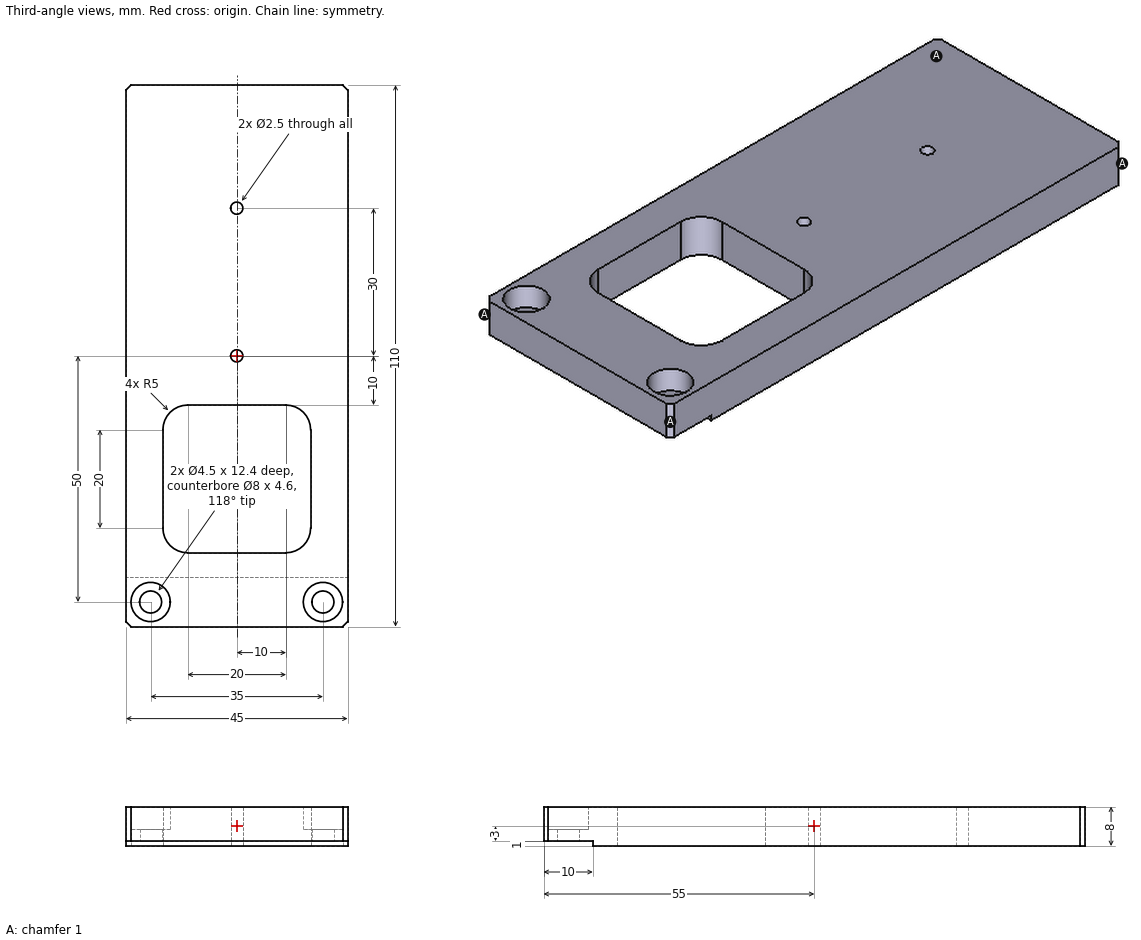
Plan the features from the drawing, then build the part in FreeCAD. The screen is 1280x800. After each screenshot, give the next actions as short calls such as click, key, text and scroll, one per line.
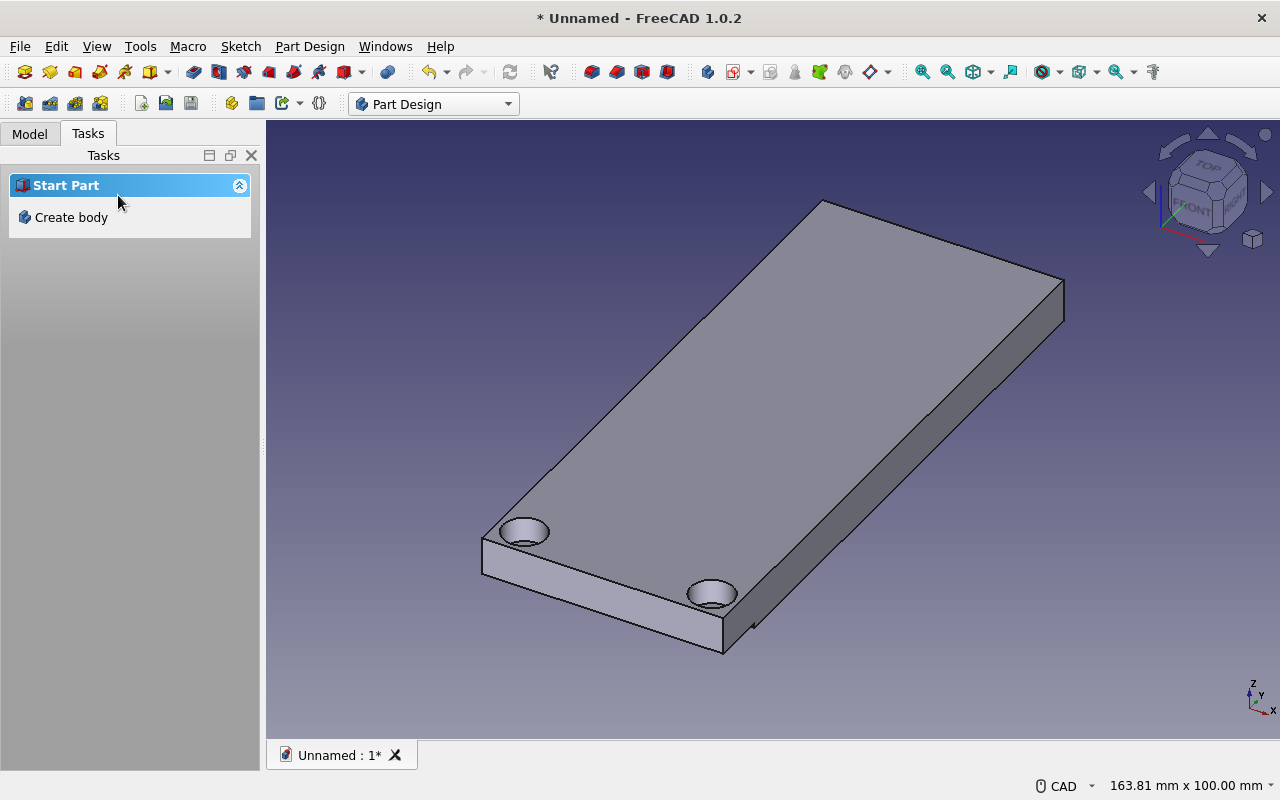
click(870, 312)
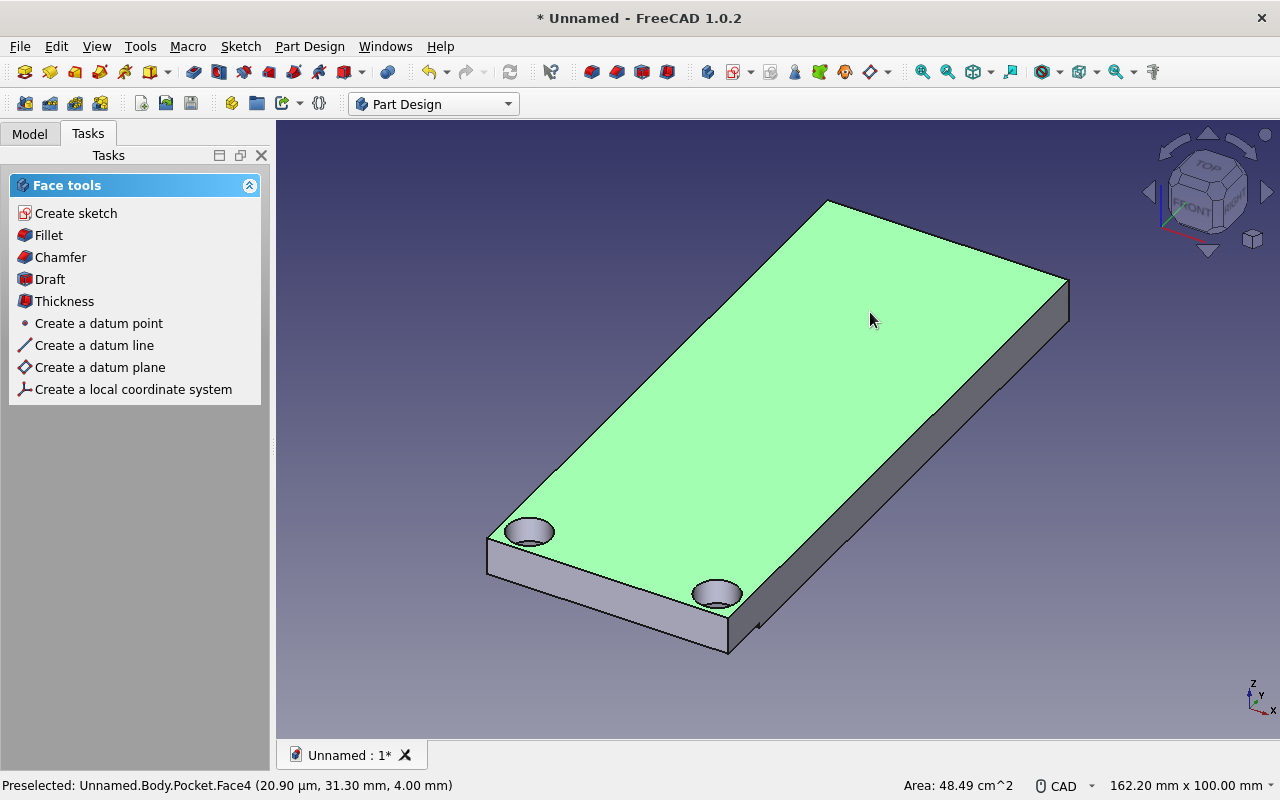
click(732, 72)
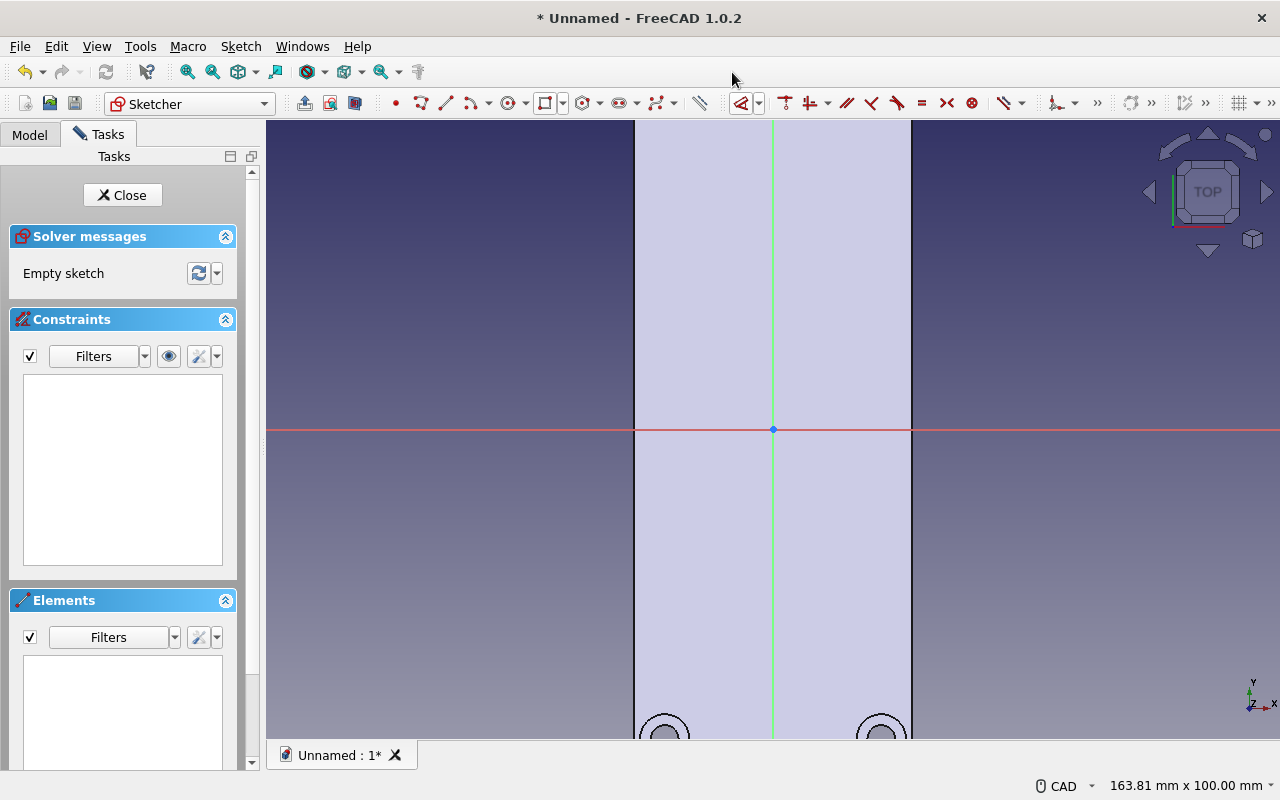
scroll(856, 224, up, 3)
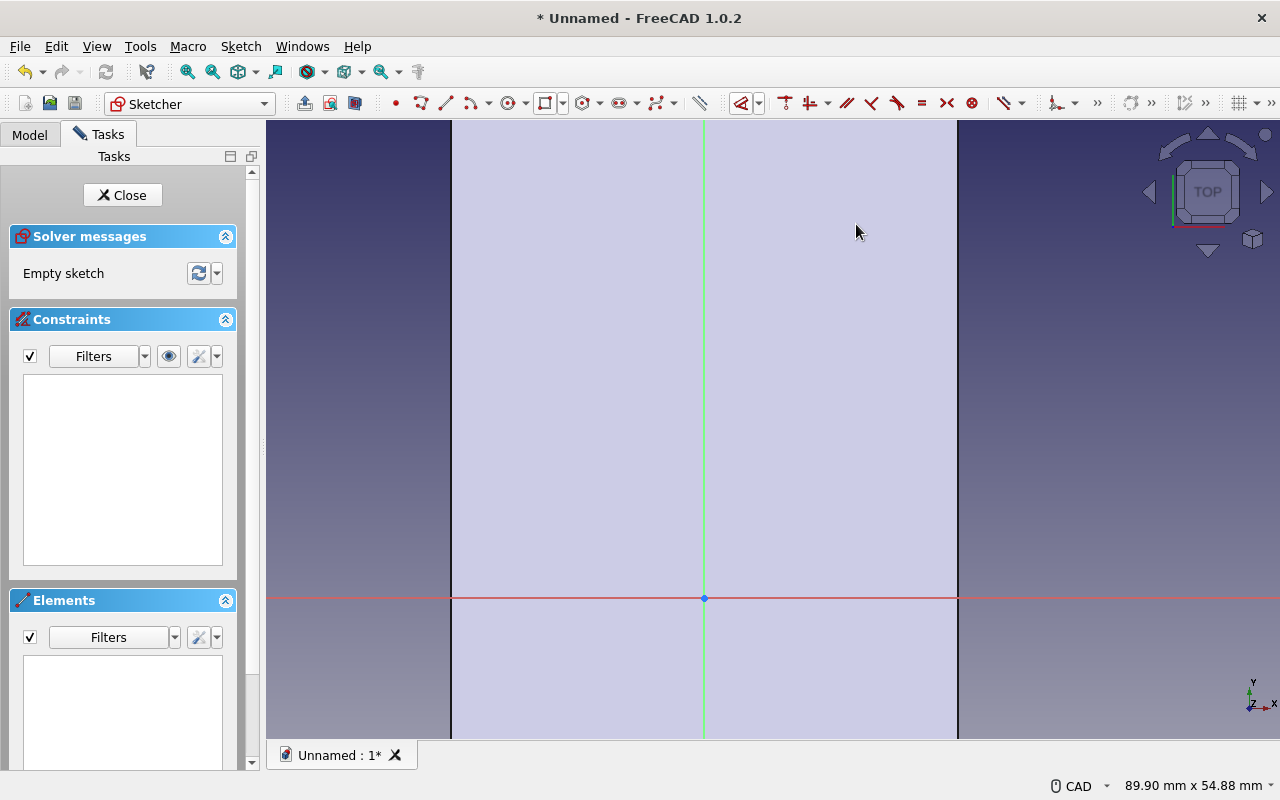
click(508, 104)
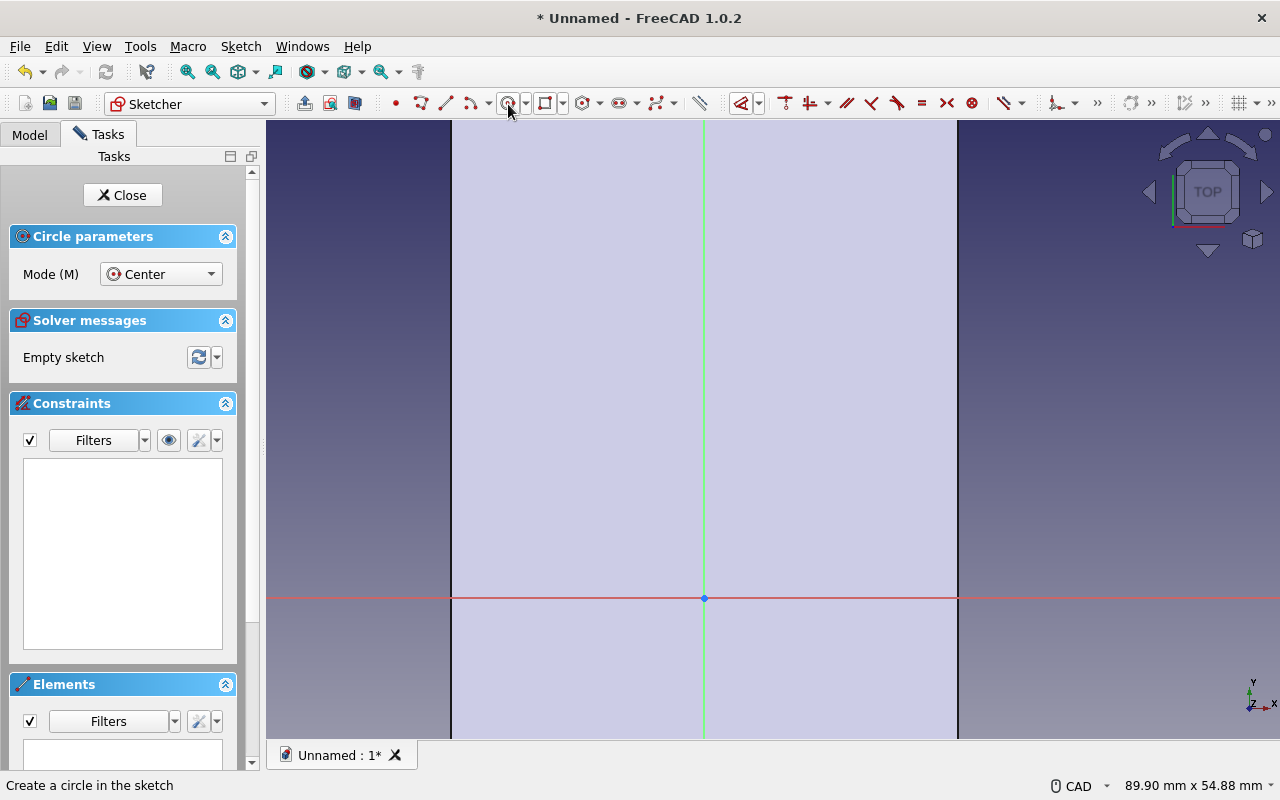
scroll(704, 260, up, 3)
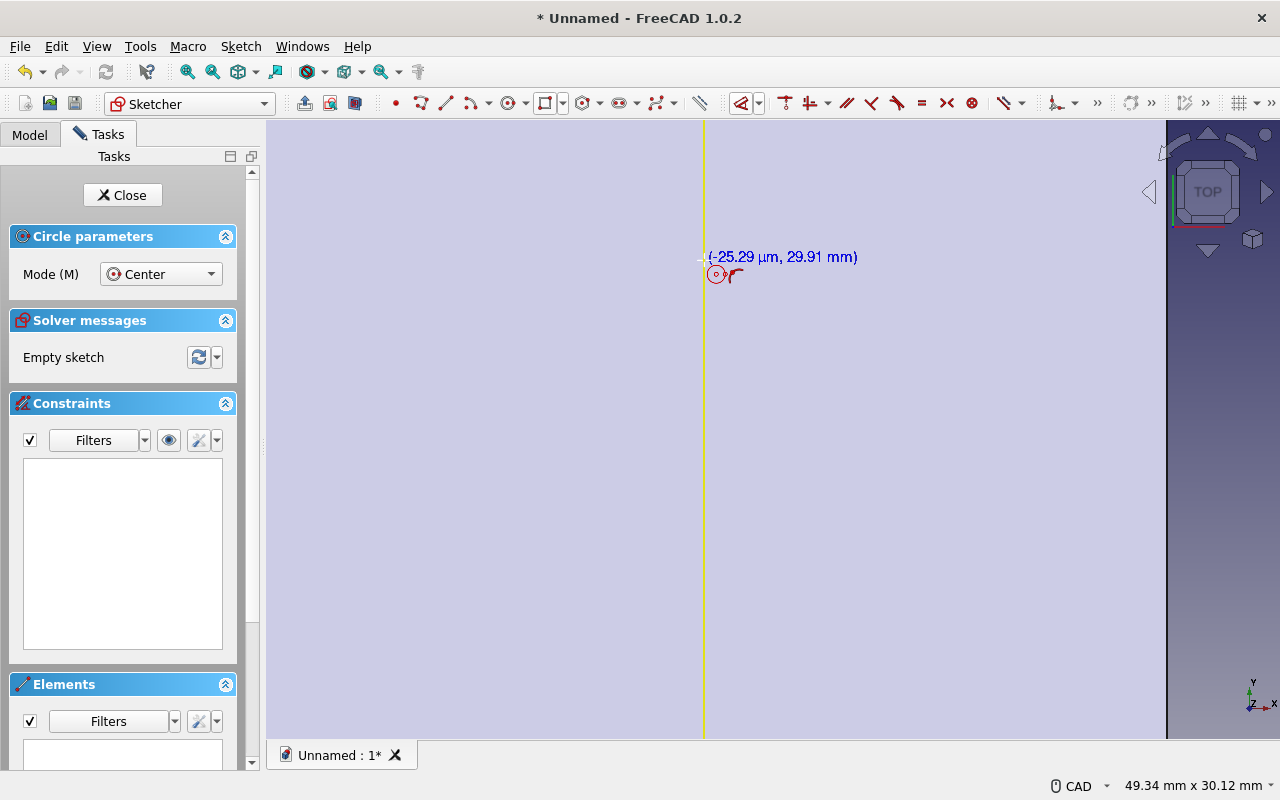
click(704, 260)
move(722, 242)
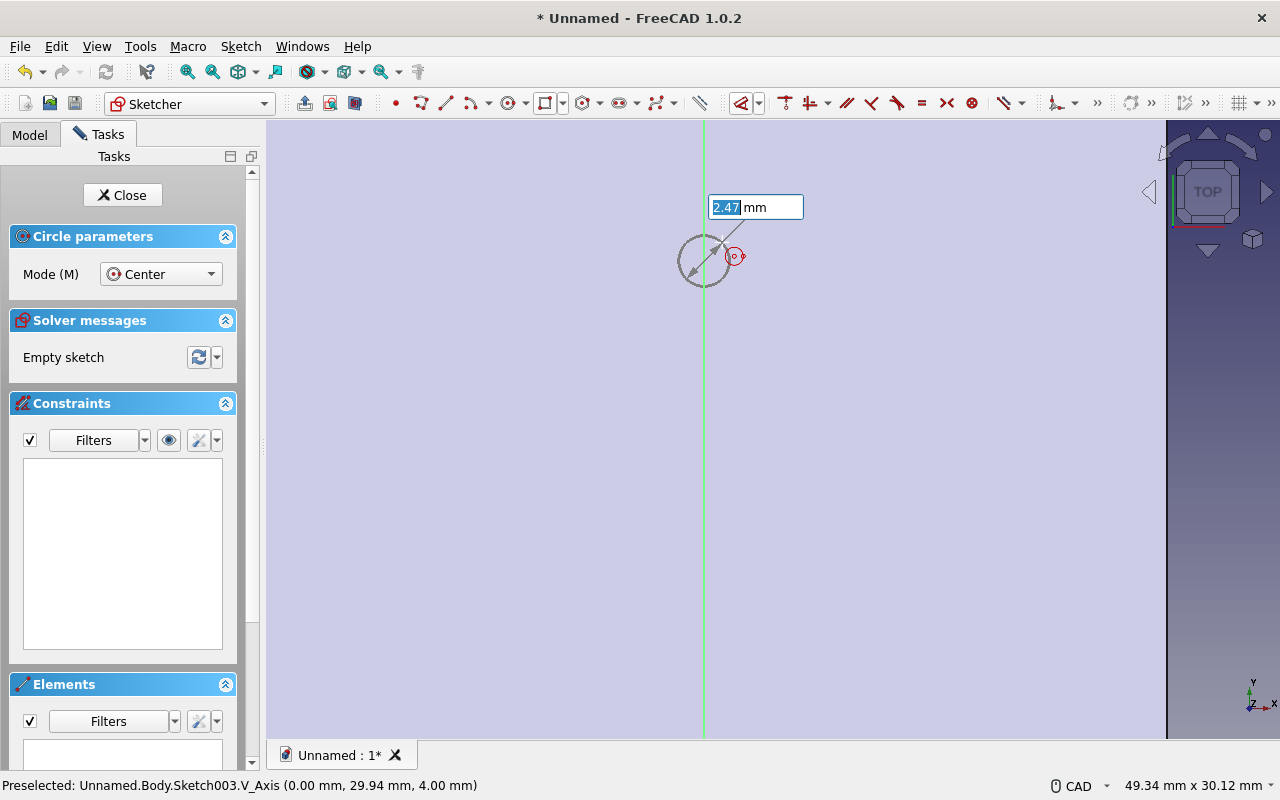
text(2.5)
key(Return)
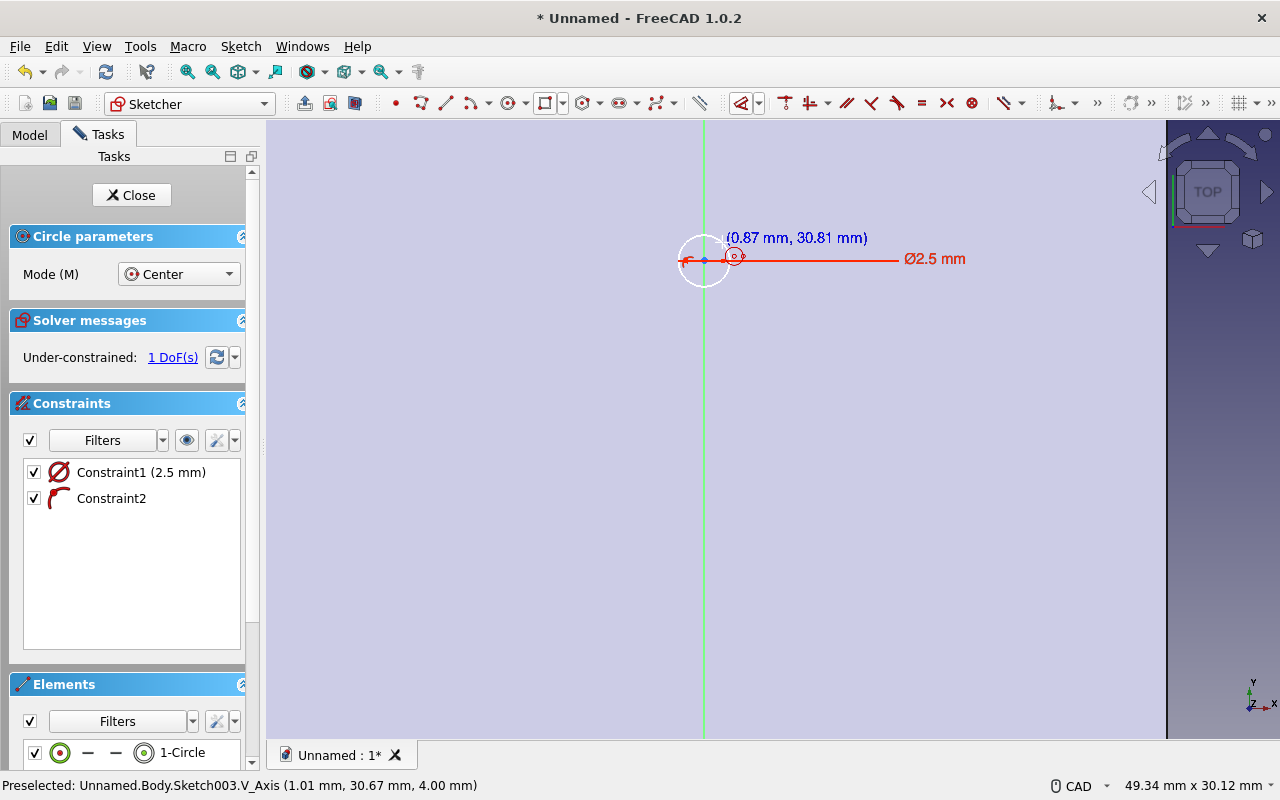
scroll(705, 261, down, 3)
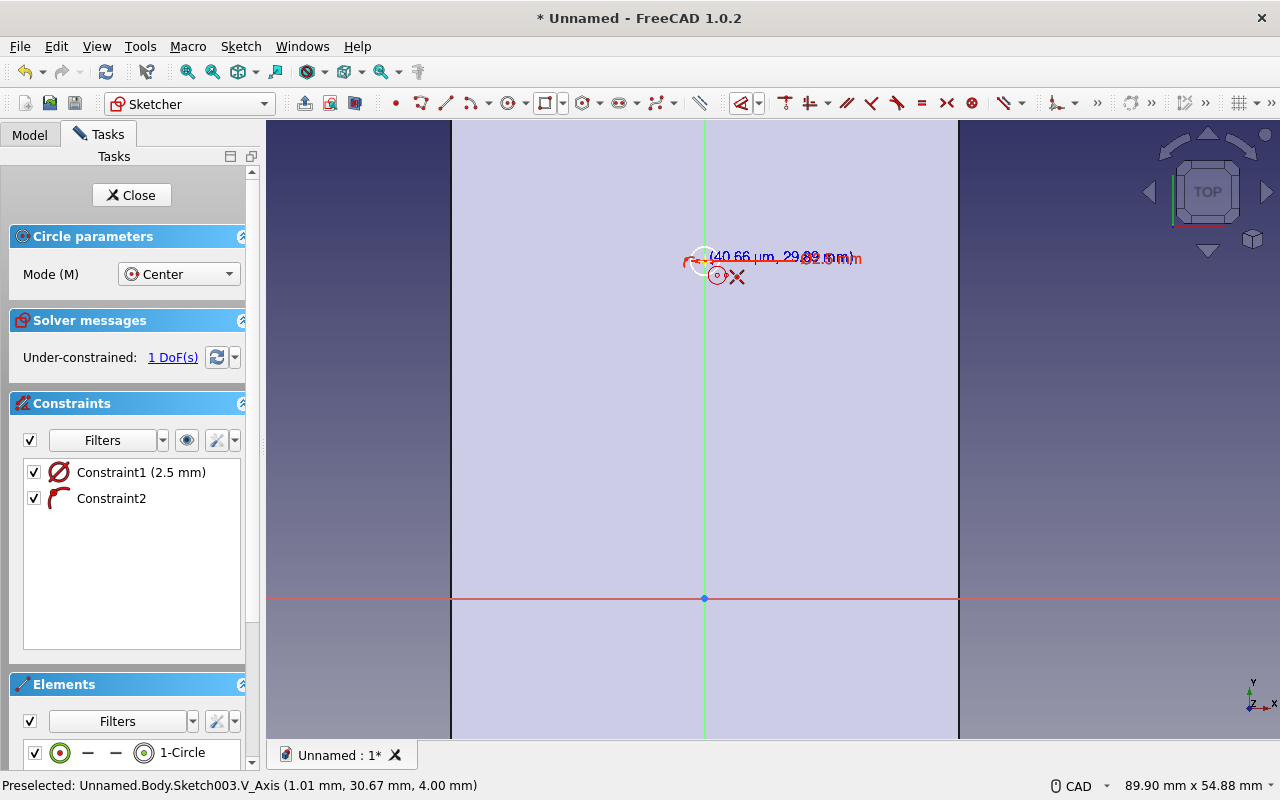
scroll(705, 599, up, 3)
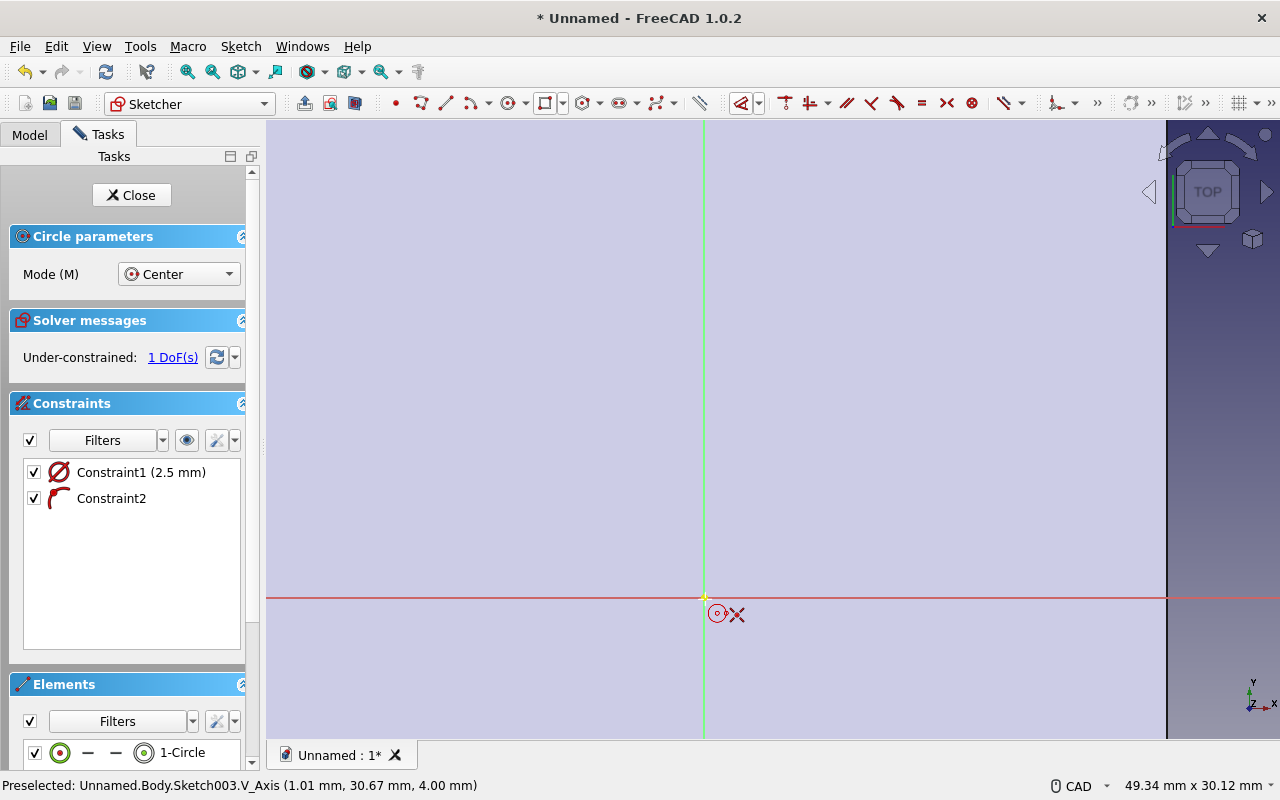
click(704, 598)
move(722, 580)